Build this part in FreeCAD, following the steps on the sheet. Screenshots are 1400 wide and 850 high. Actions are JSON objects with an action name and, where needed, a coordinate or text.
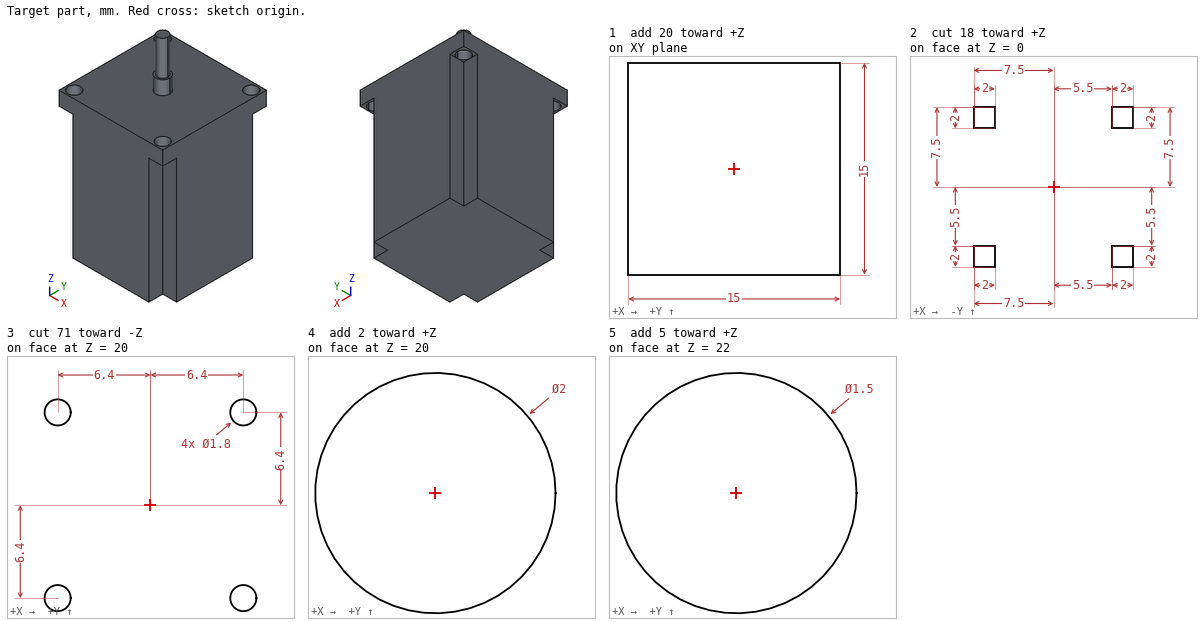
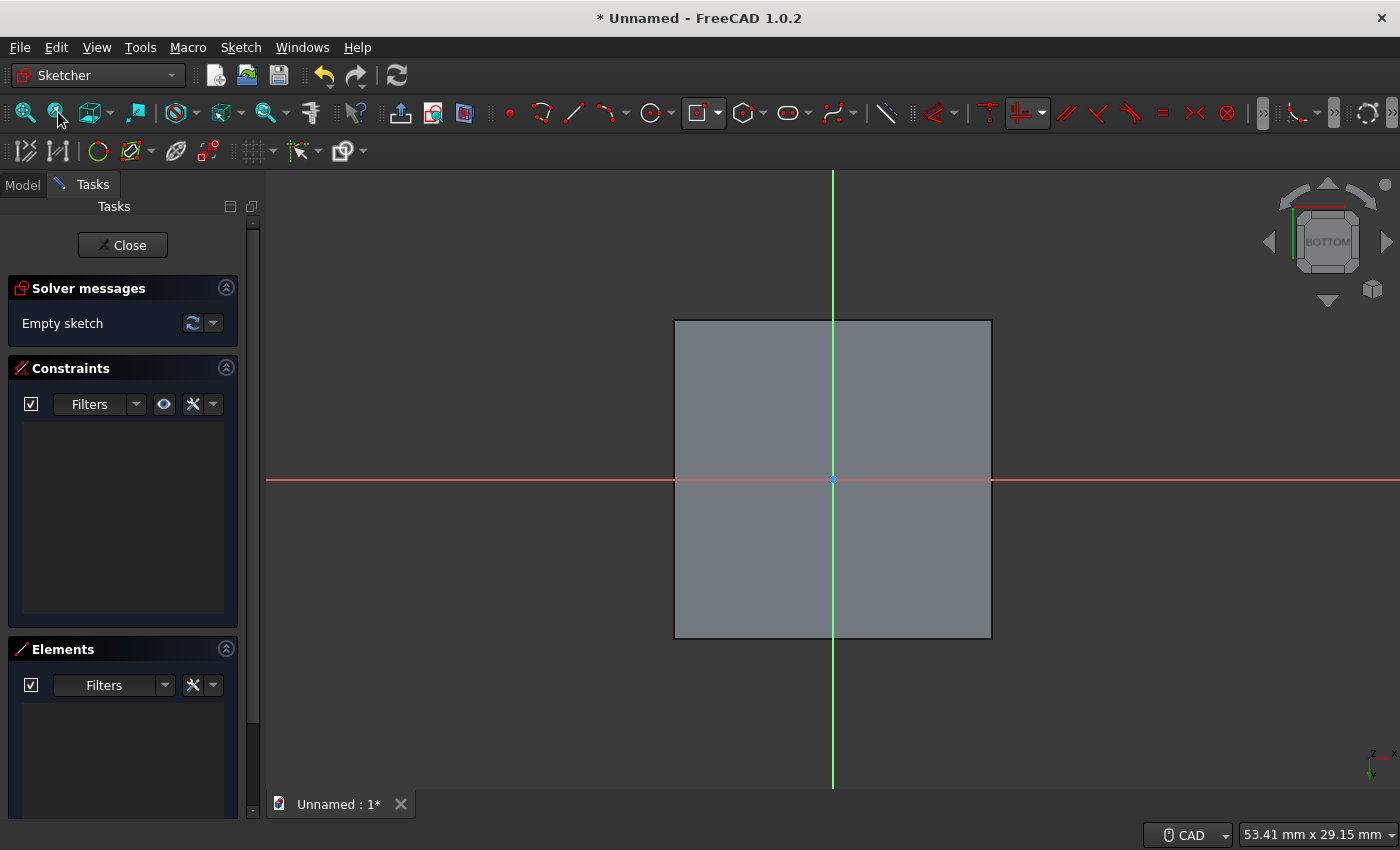
{"action": "key", "text": "g r"}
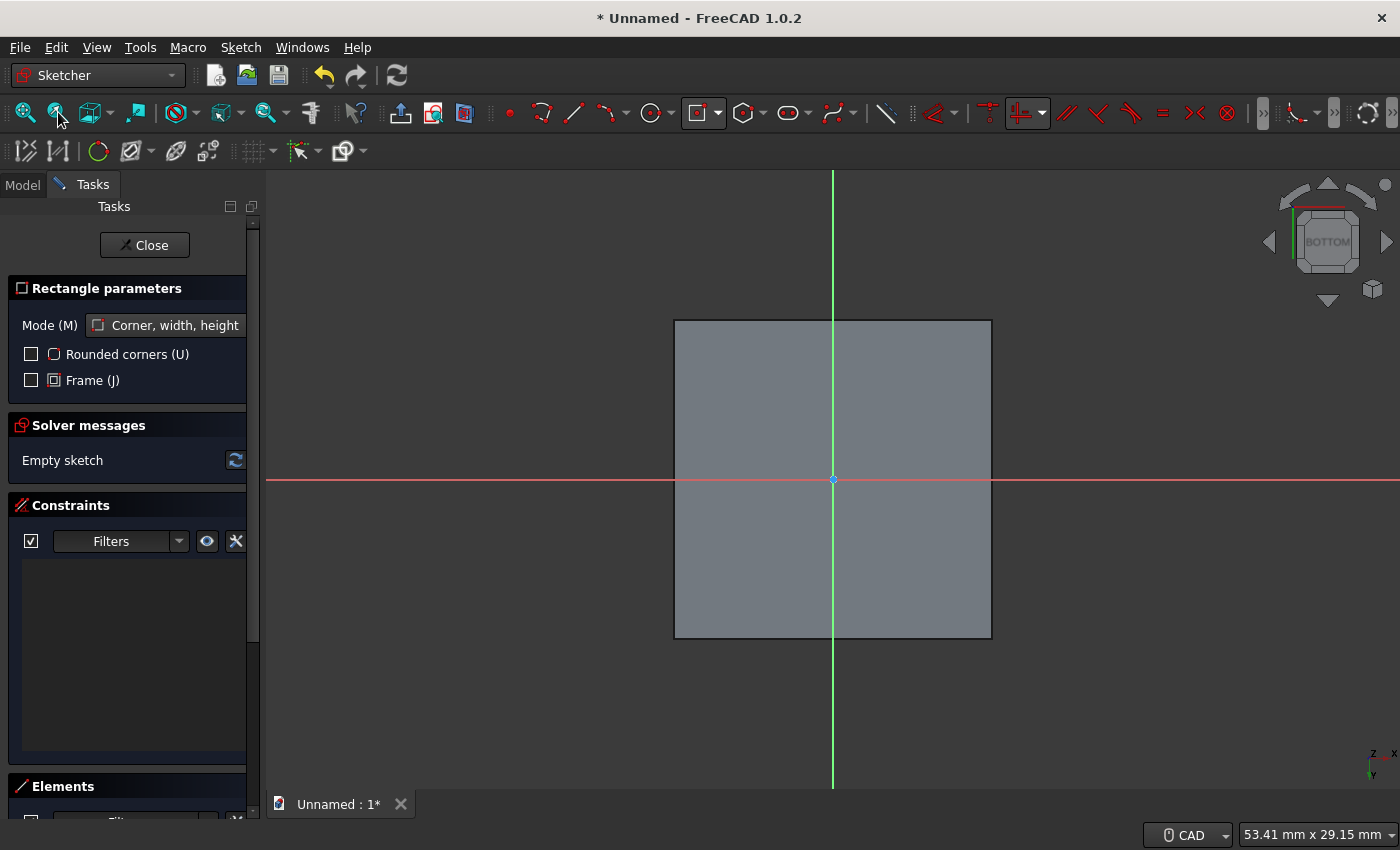
{"action": "left_click", "coordinate": [674, 596]}
{"action": "mouse_move", "coordinate": [716, 639]}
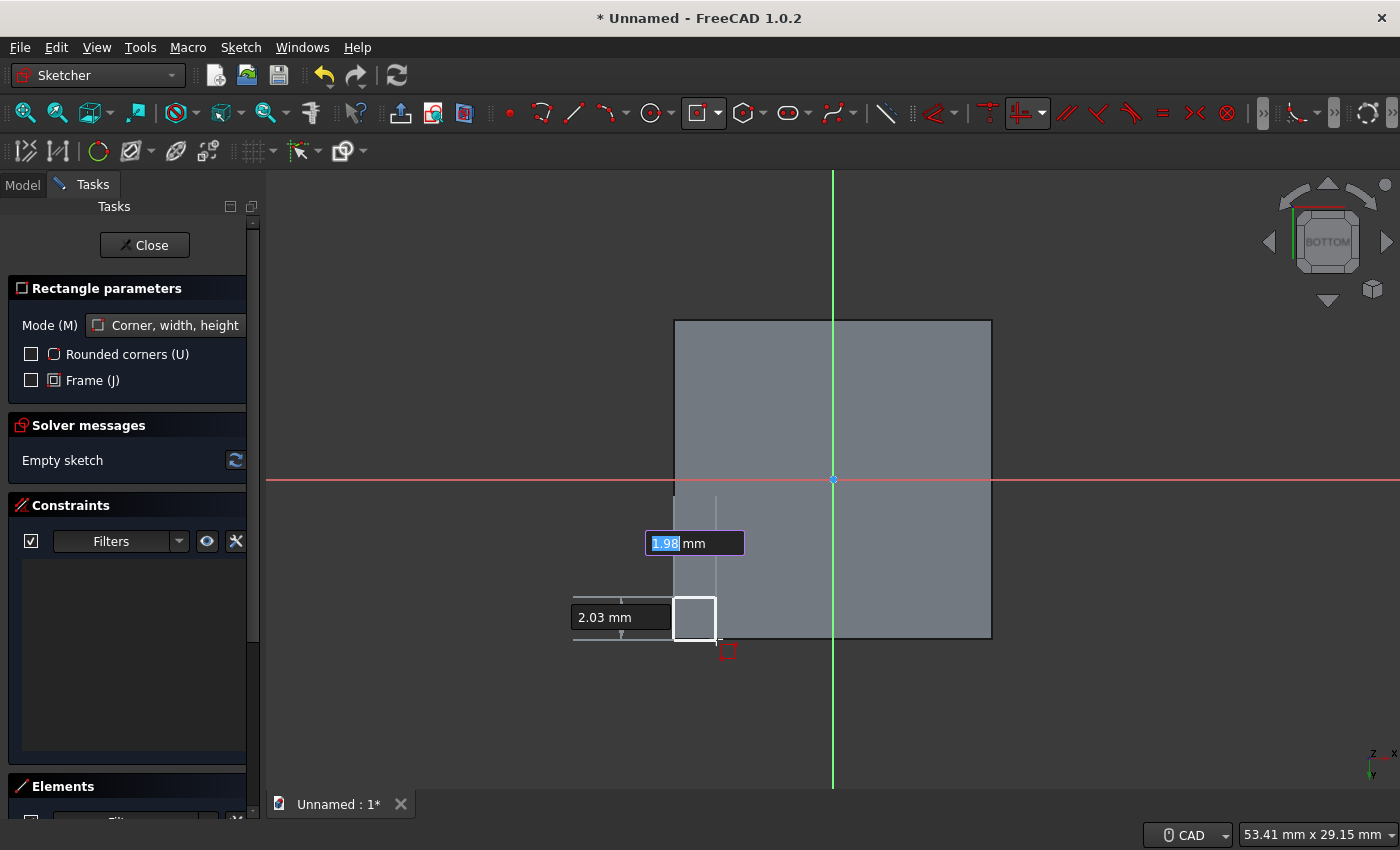
{"action": "type", "text": "2"}
{"action": "key", "text": "Tab"}
{"action": "type", "text": "2"}
{"action": "key", "text": "Return"}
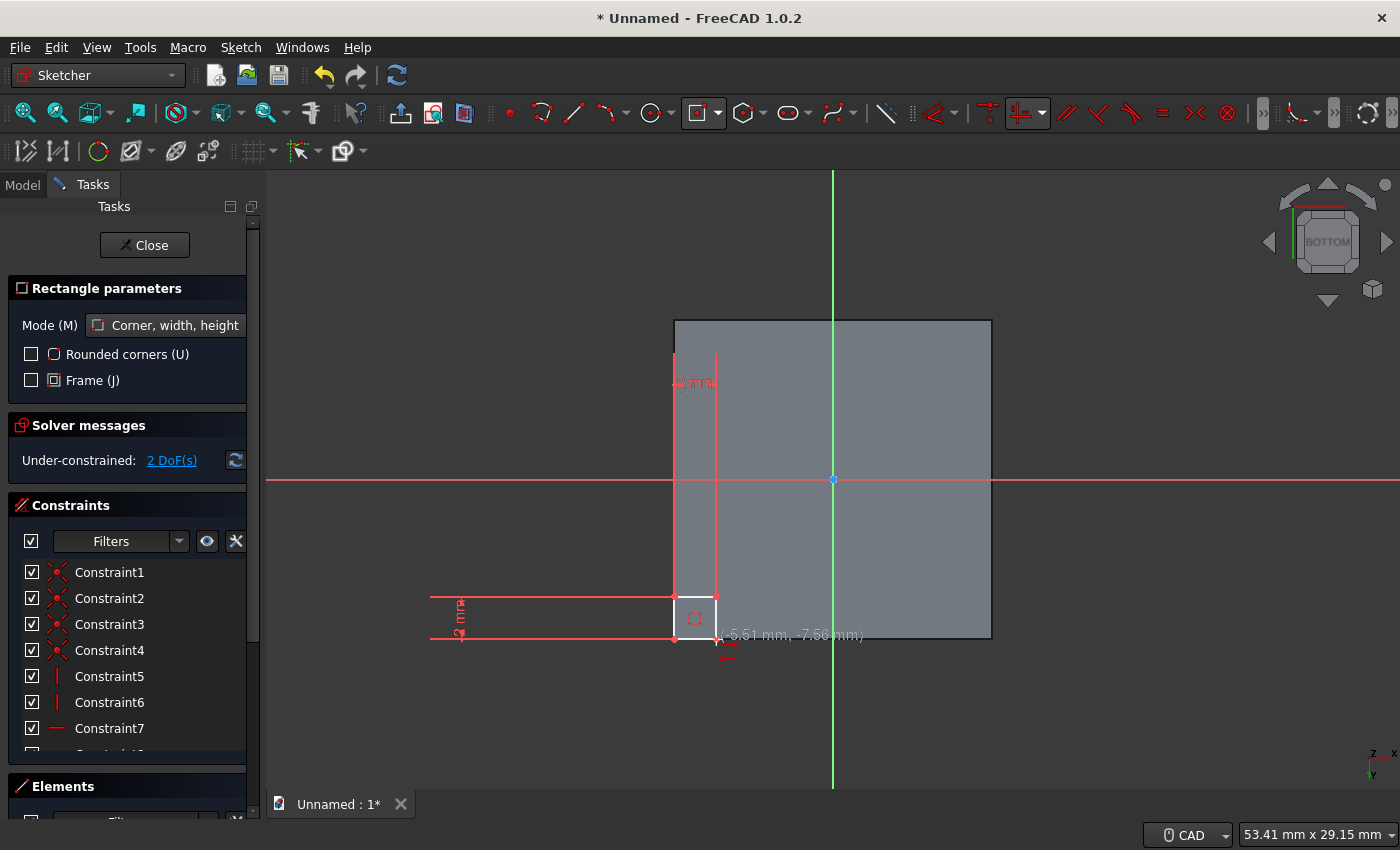
{"action": "left_click", "coordinate": [674, 320]}
{"action": "mouse_move", "coordinate": [716, 363]}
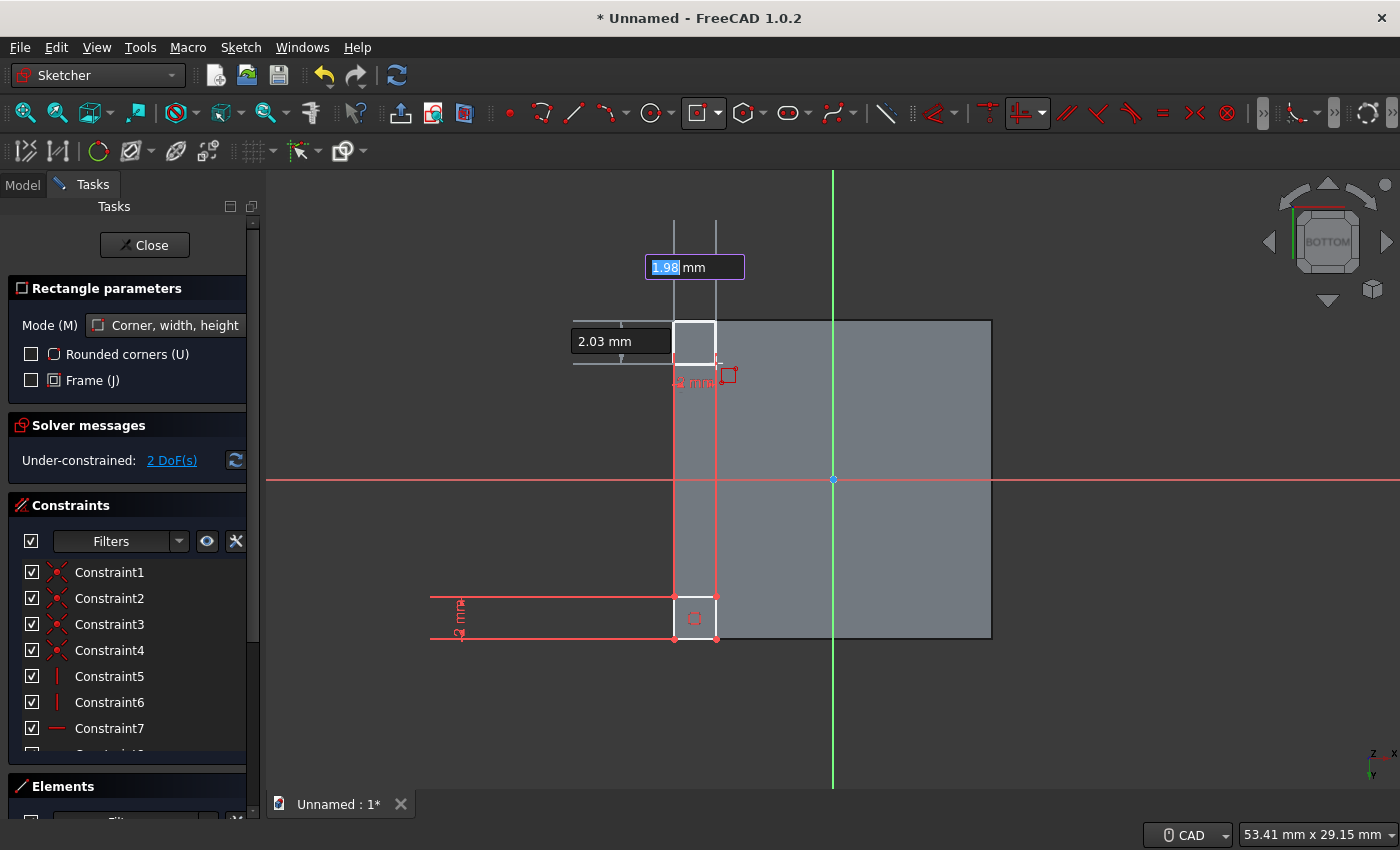
{"action": "type", "text": "2"}
{"action": "key", "text": "Tab"}
{"action": "type", "text": "2"}
{"action": "key", "text": "Return"}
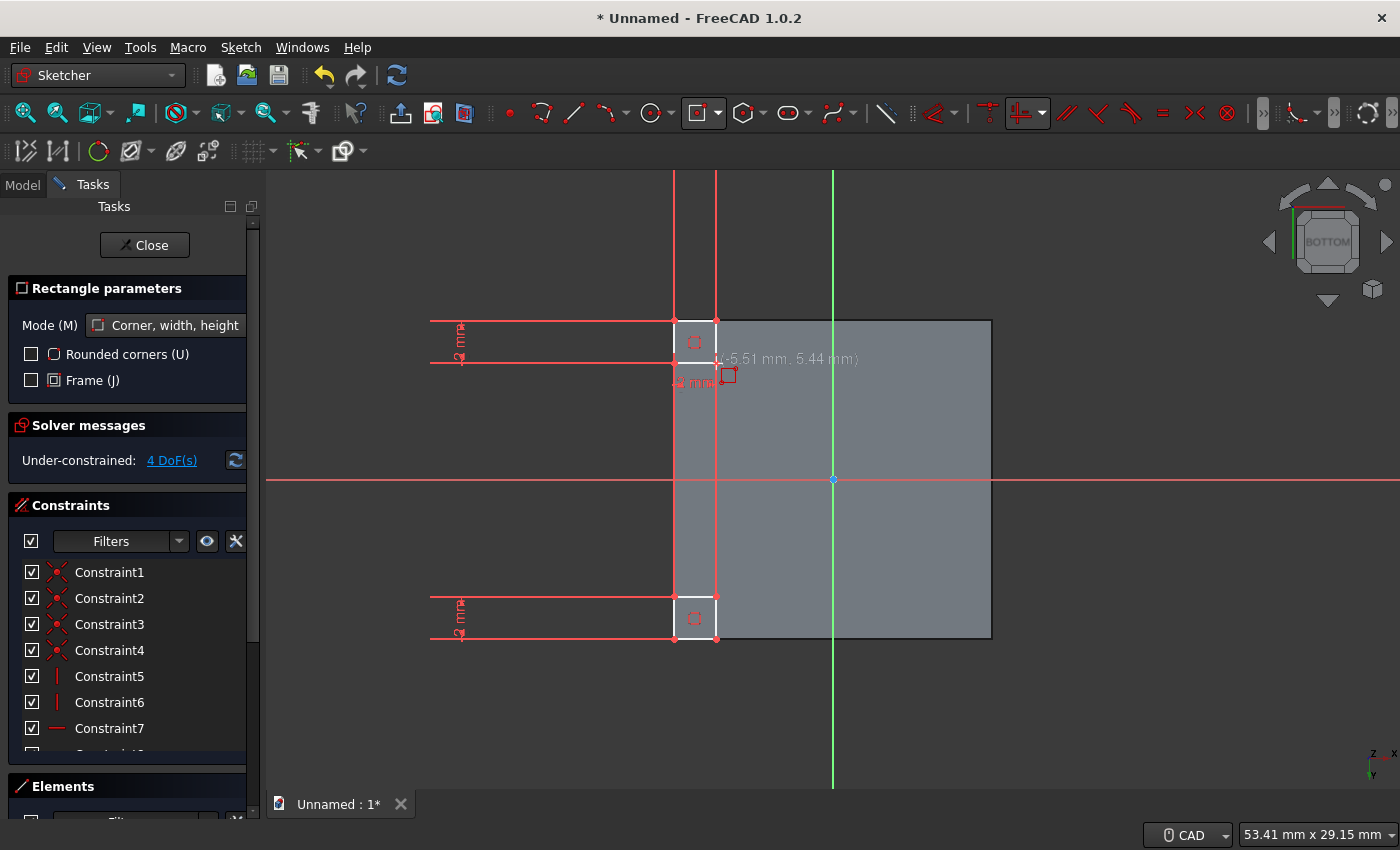
{"action": "left_click", "coordinate": [950, 320]}
{"action": "mouse_move", "coordinate": [992, 363]}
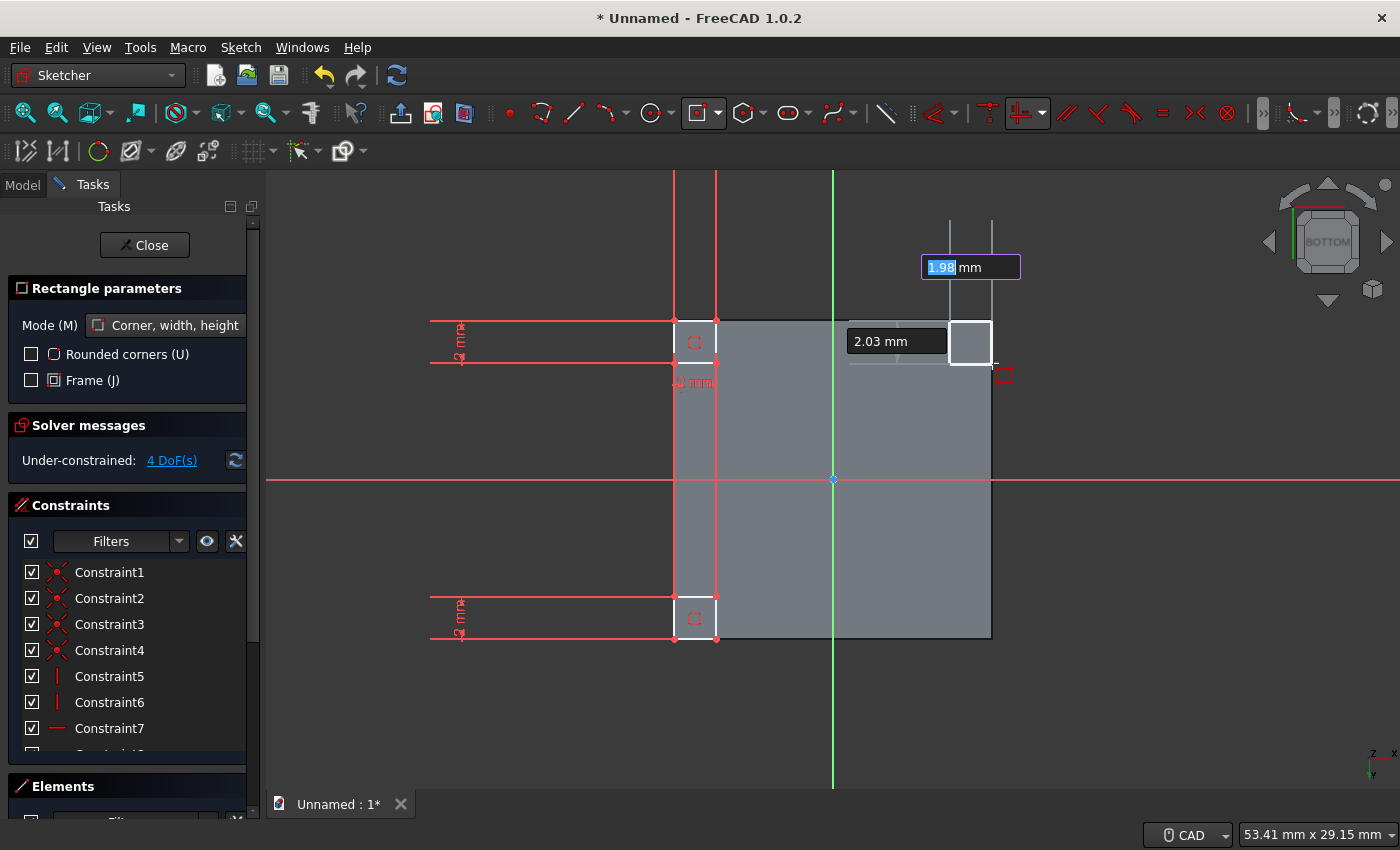
{"action": "type", "text": "2"}
{"action": "key", "text": "Tab"}
{"action": "type", "text": "2"}
{"action": "key", "text": "Return"}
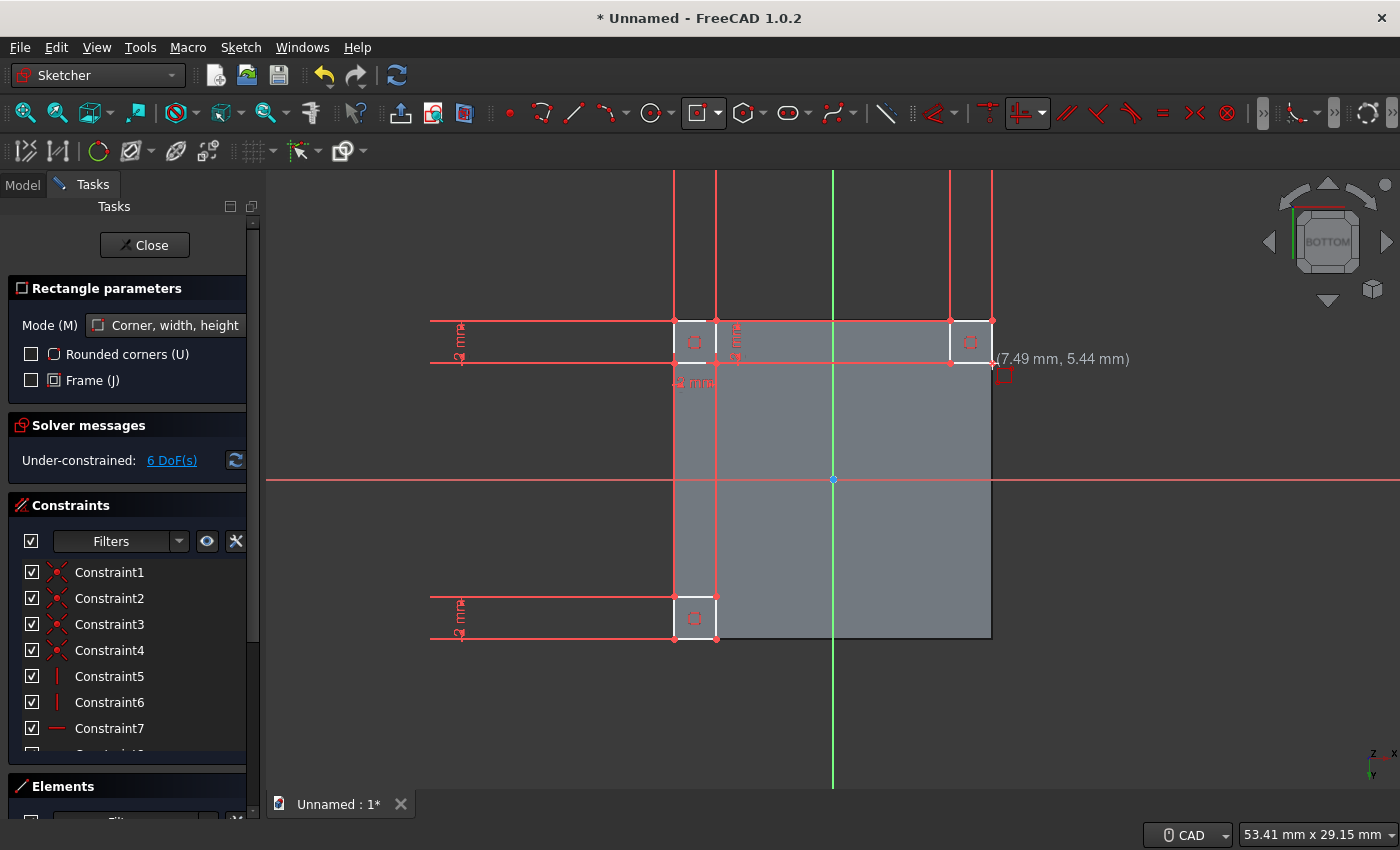
{"action": "left_click", "coordinate": [950, 596]}
{"action": "mouse_move", "coordinate": [992, 639]}